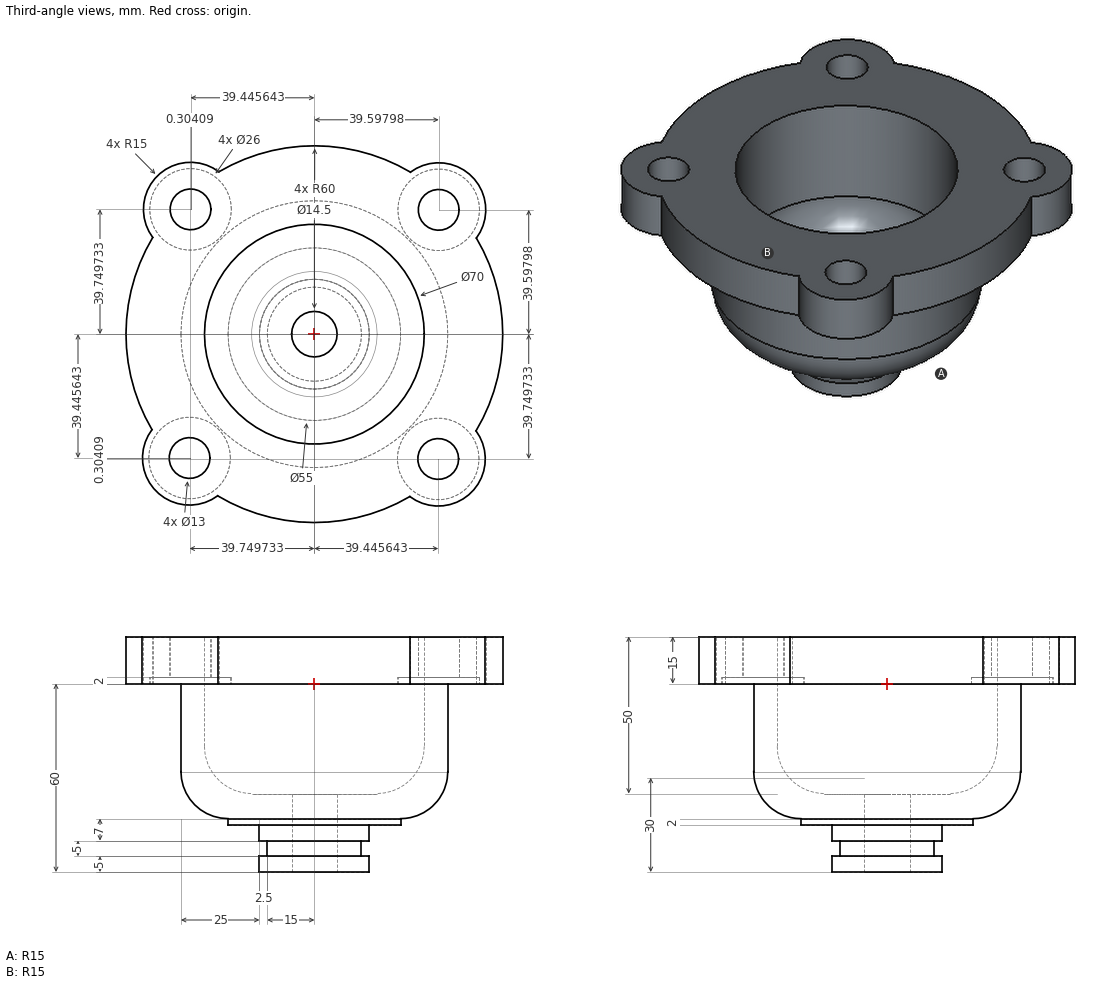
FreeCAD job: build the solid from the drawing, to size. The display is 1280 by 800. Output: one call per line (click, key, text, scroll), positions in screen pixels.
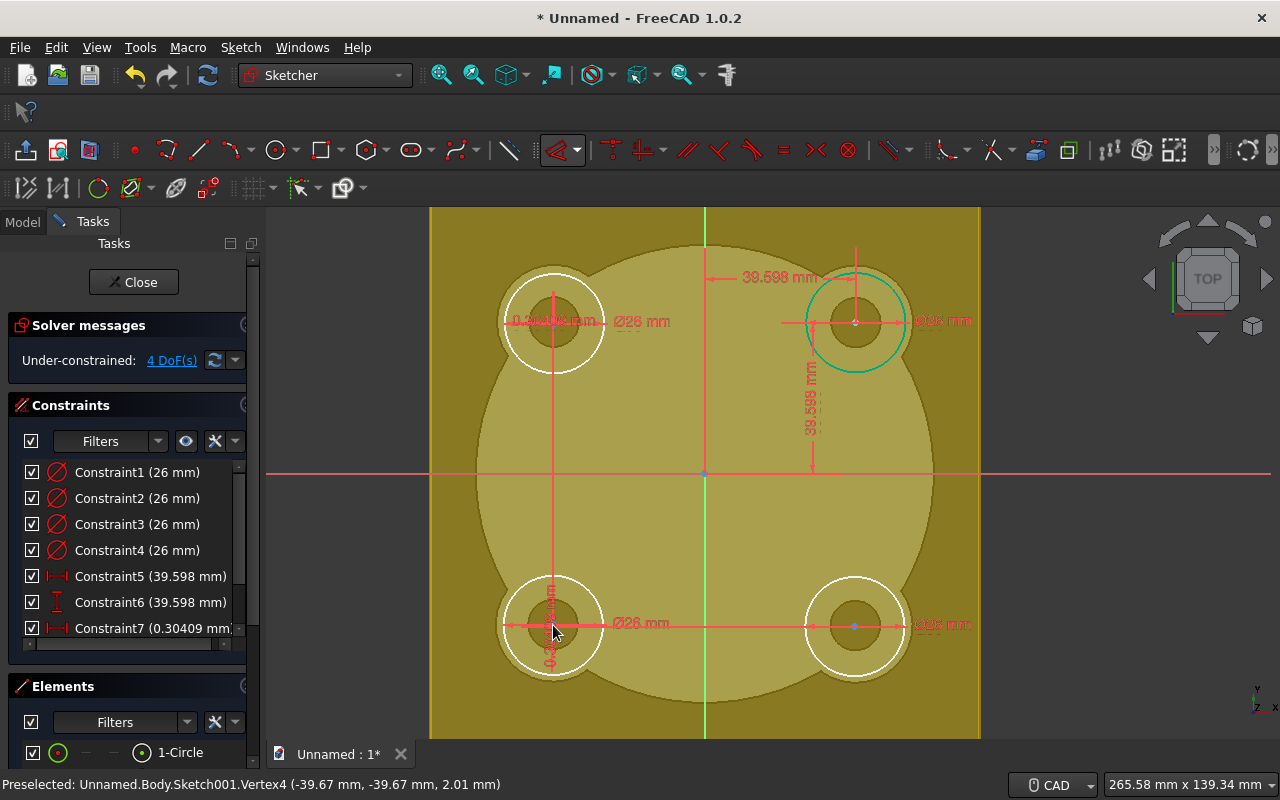
click(554, 324)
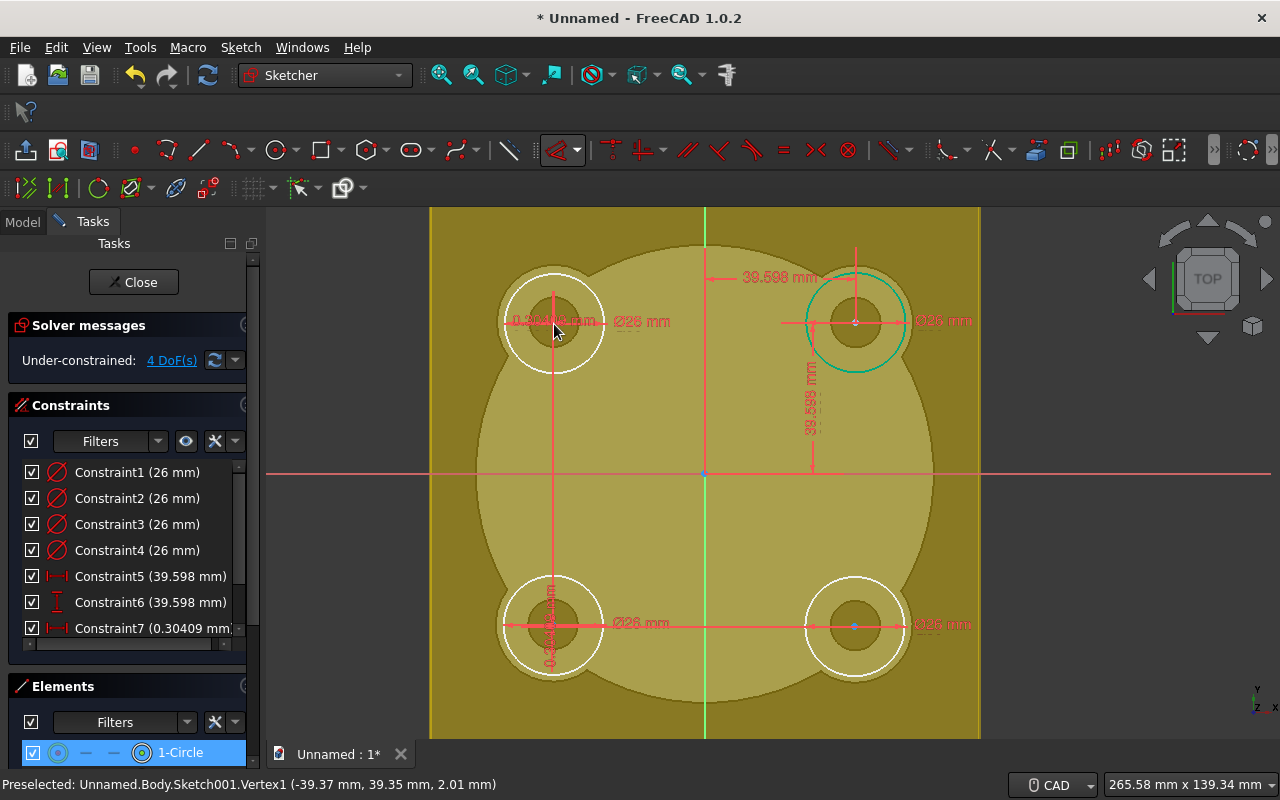
key(l)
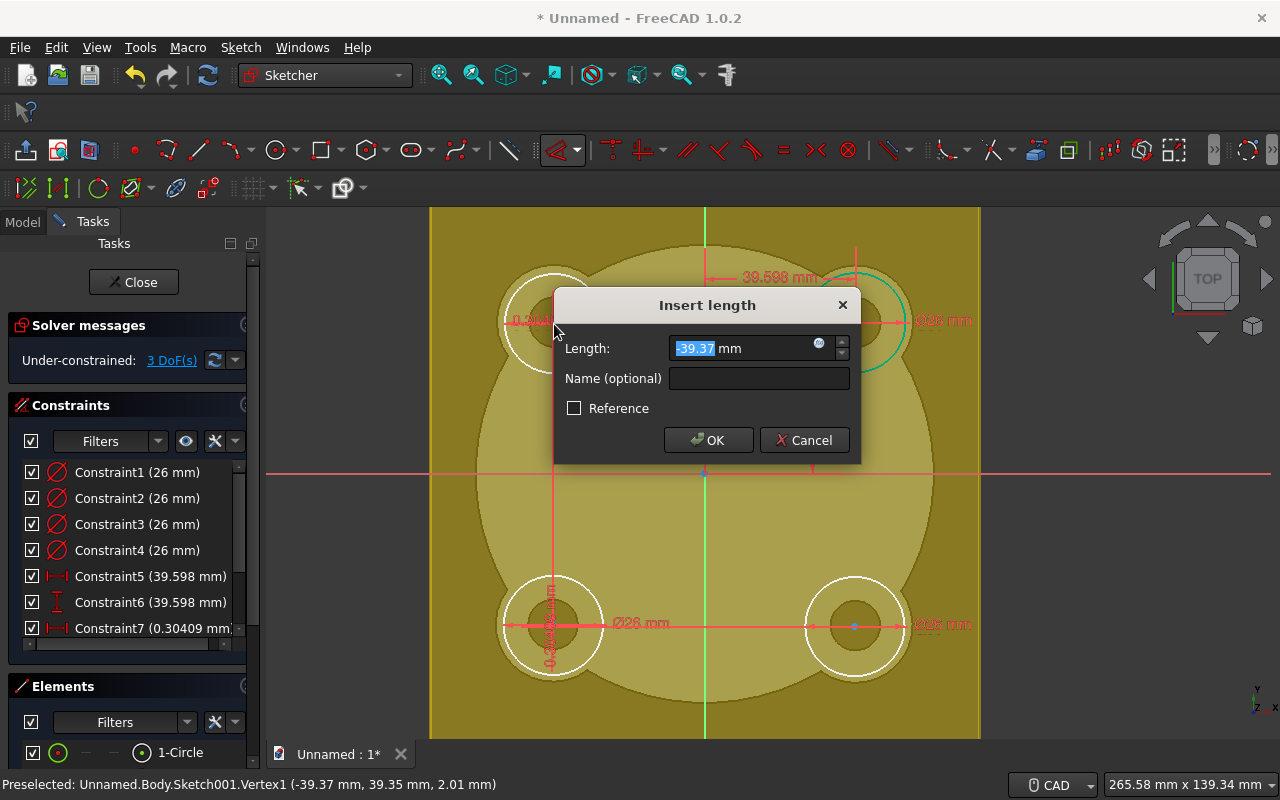
text(-39.445643)
key(Return)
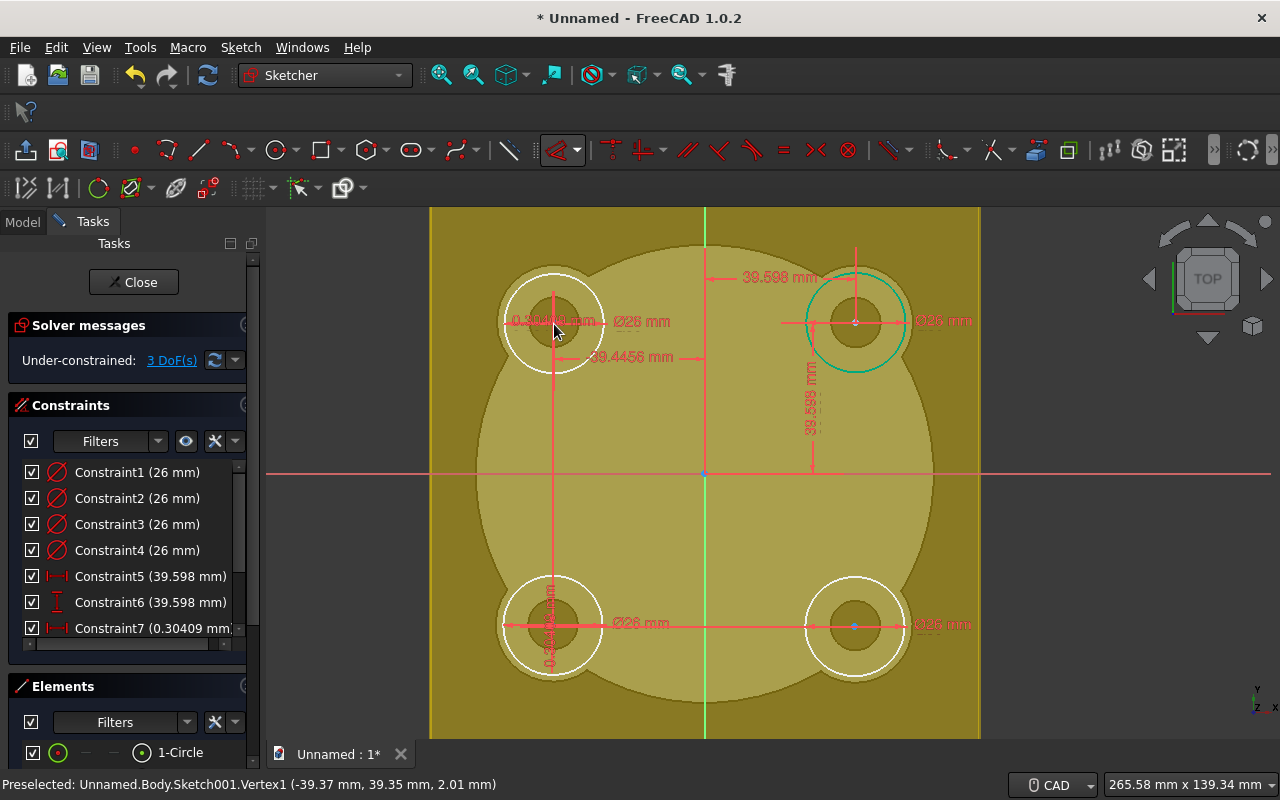
click(554, 324)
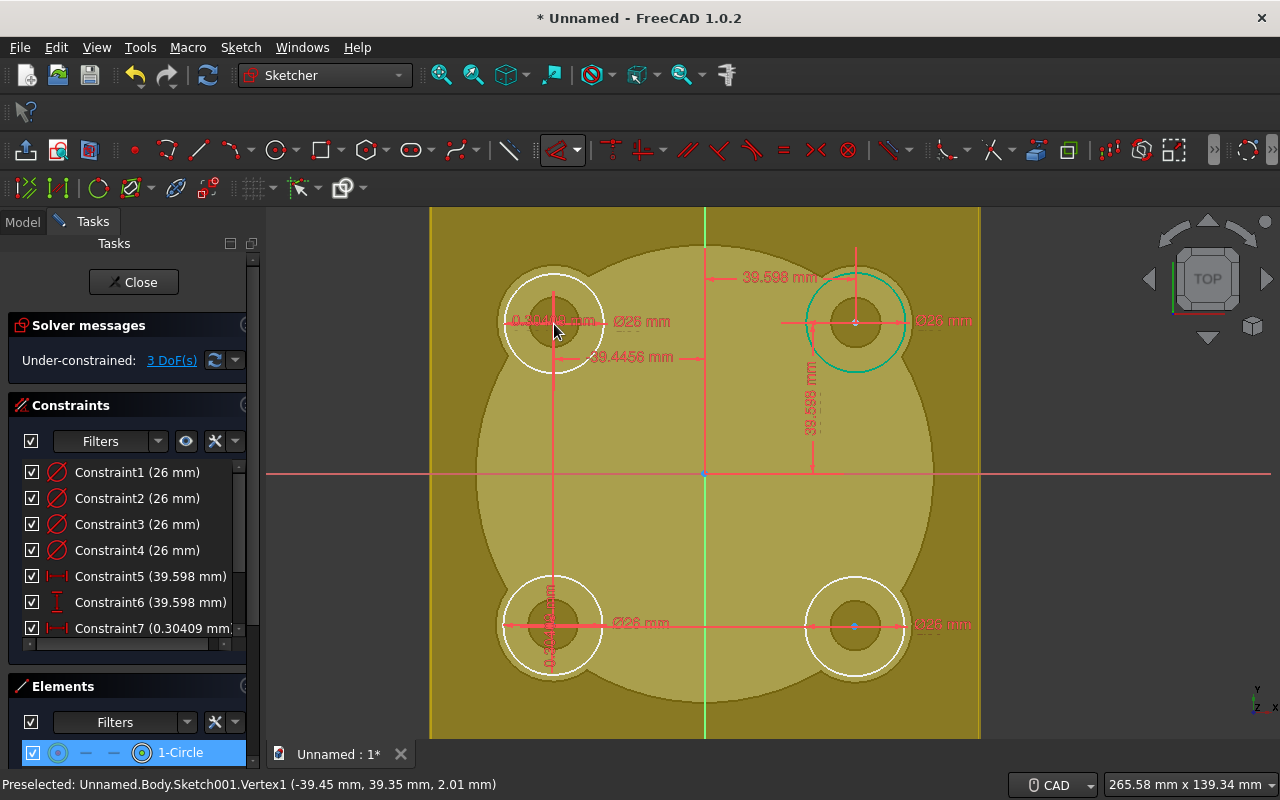
key(i)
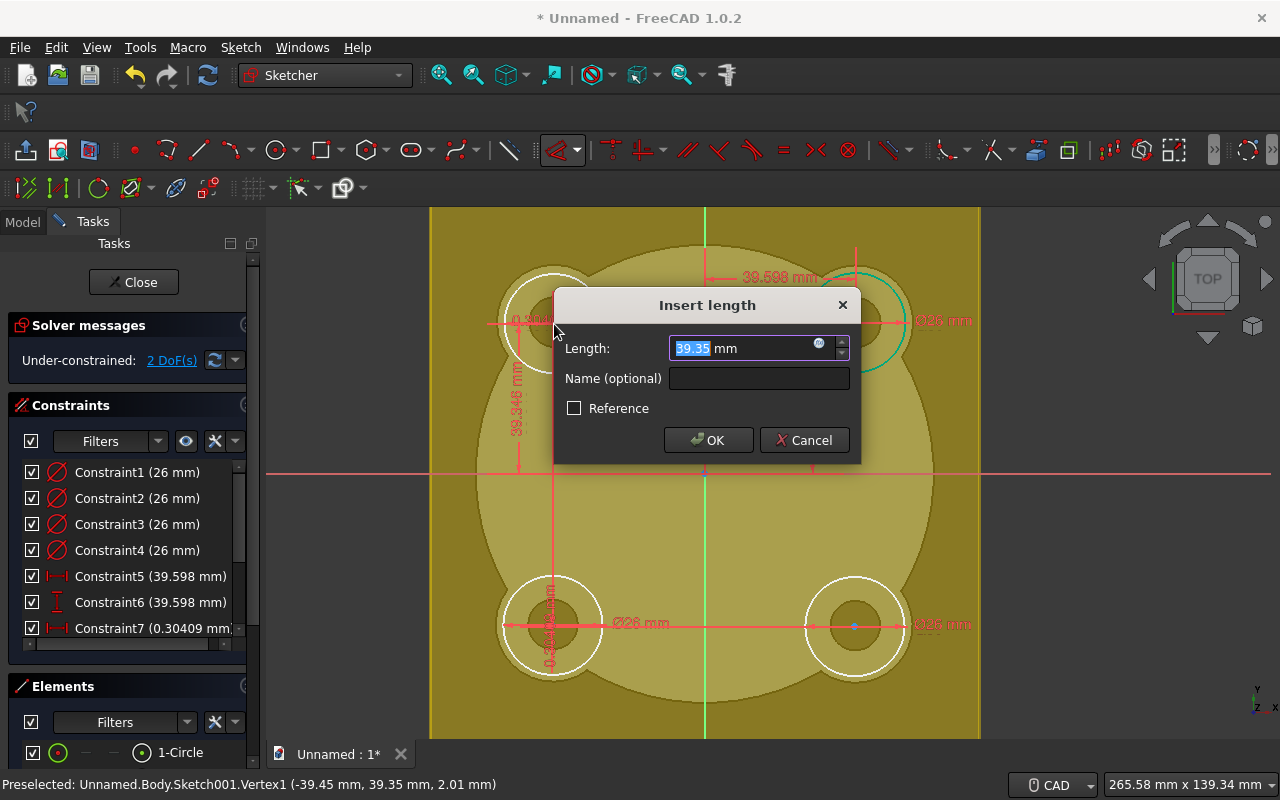
text(39.749733)
key(Return)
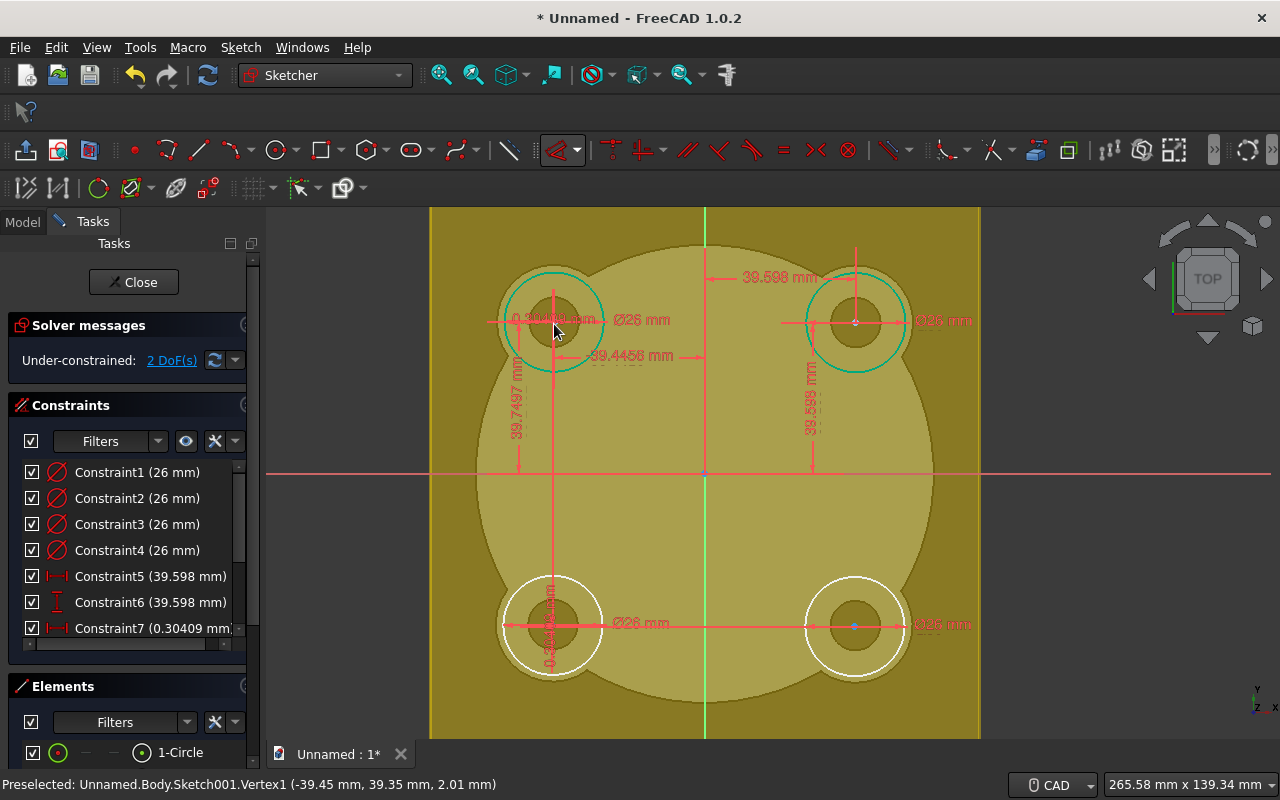
click(855, 627)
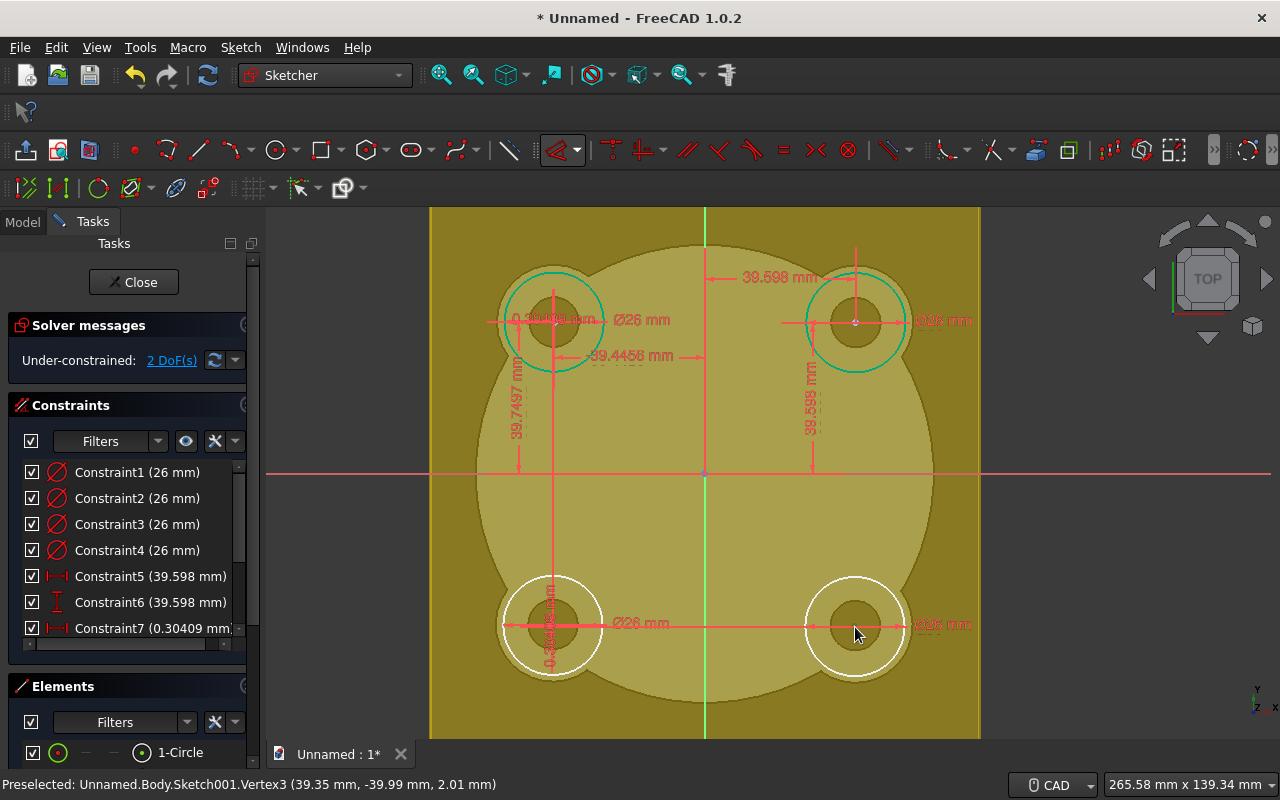
key(l)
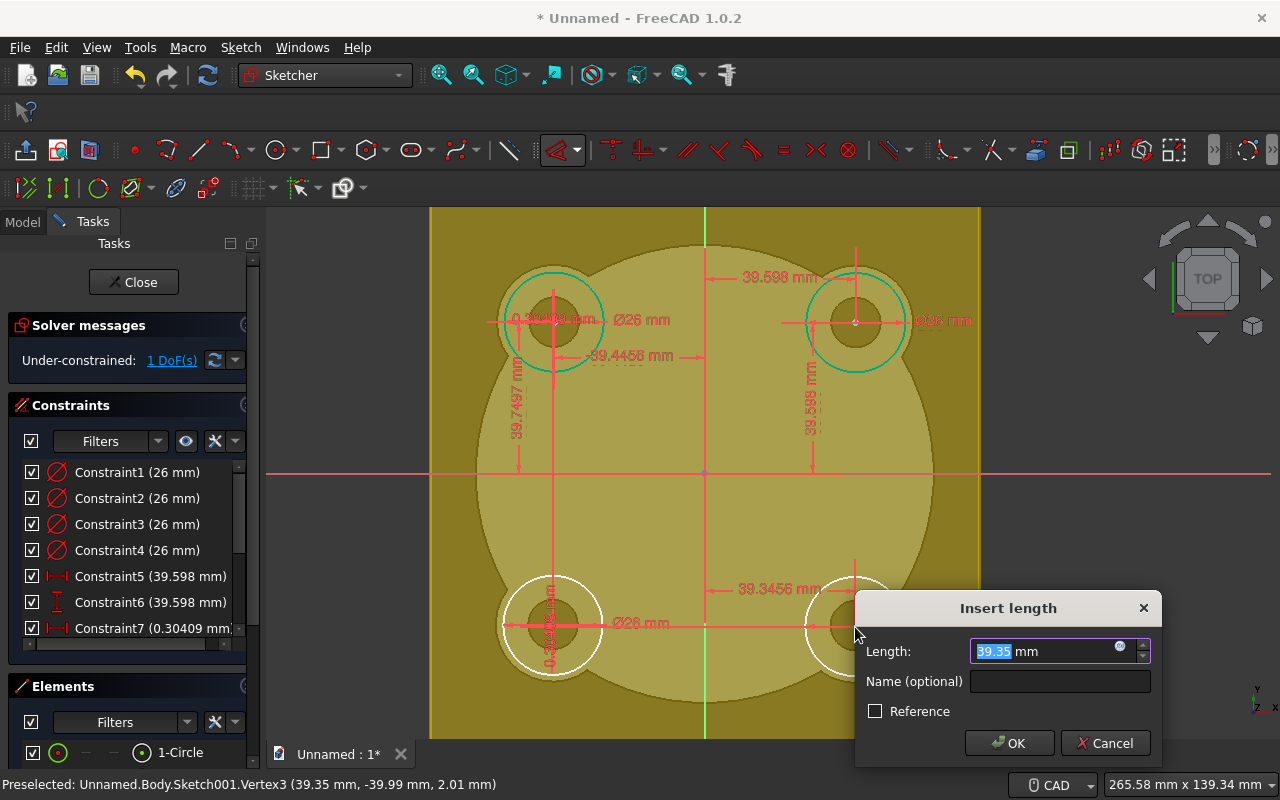
text(39.445643)
key(Return)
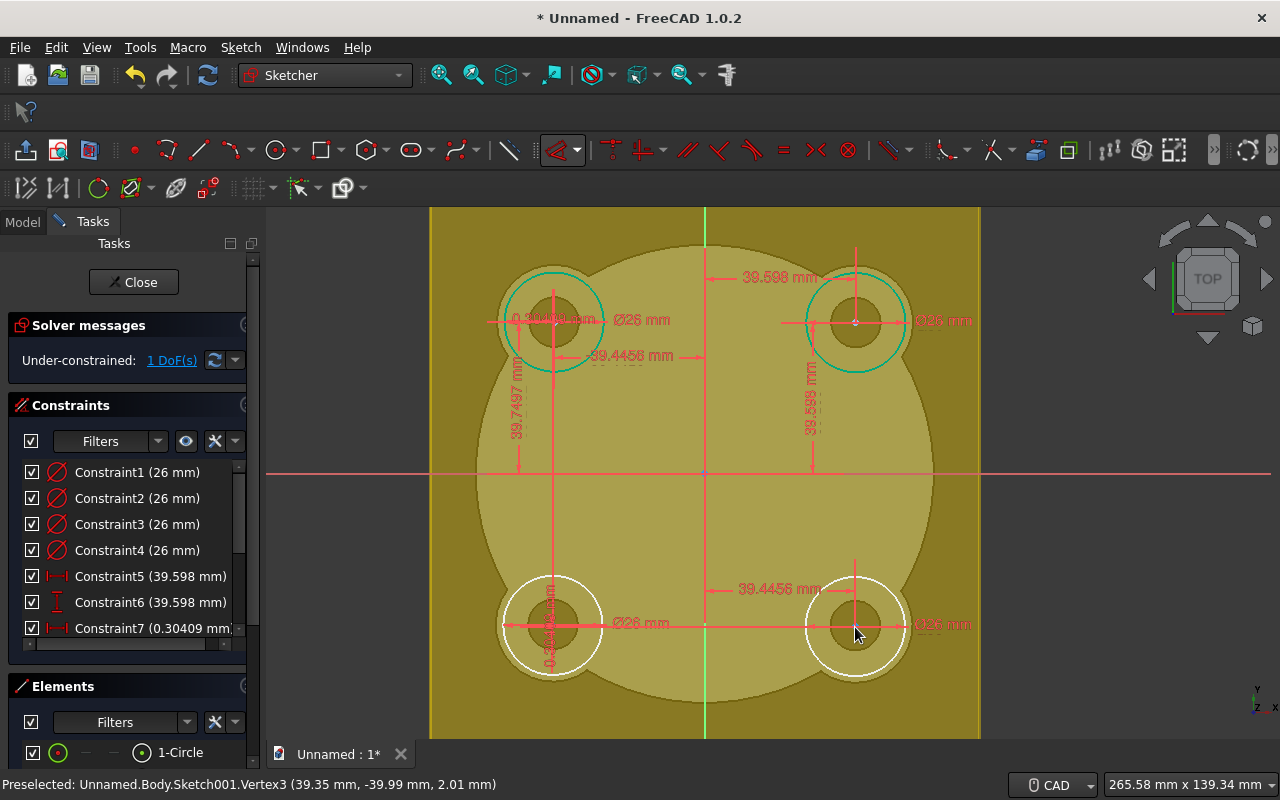
click(855, 627)